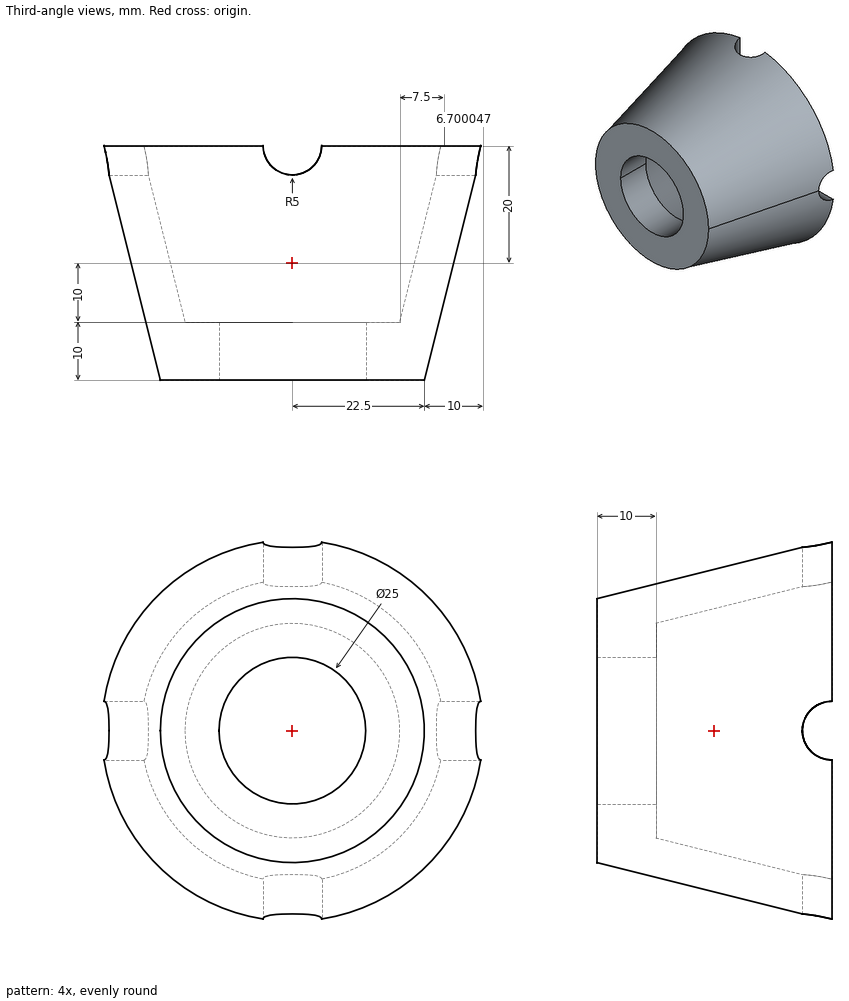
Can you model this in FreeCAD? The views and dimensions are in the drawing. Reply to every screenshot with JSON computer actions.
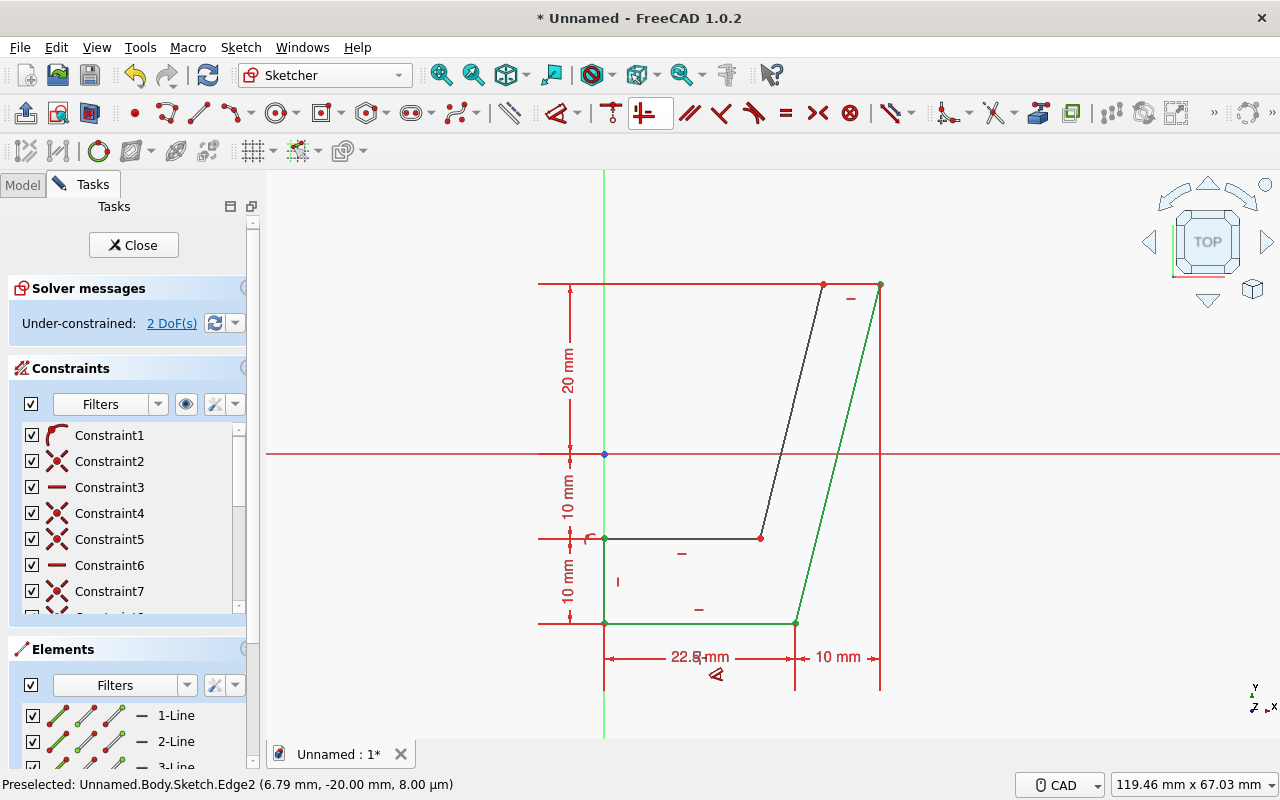
{"action": "left_click", "coordinate": [804, 361]}
{"action": "left_click", "coordinate": [792, 250]}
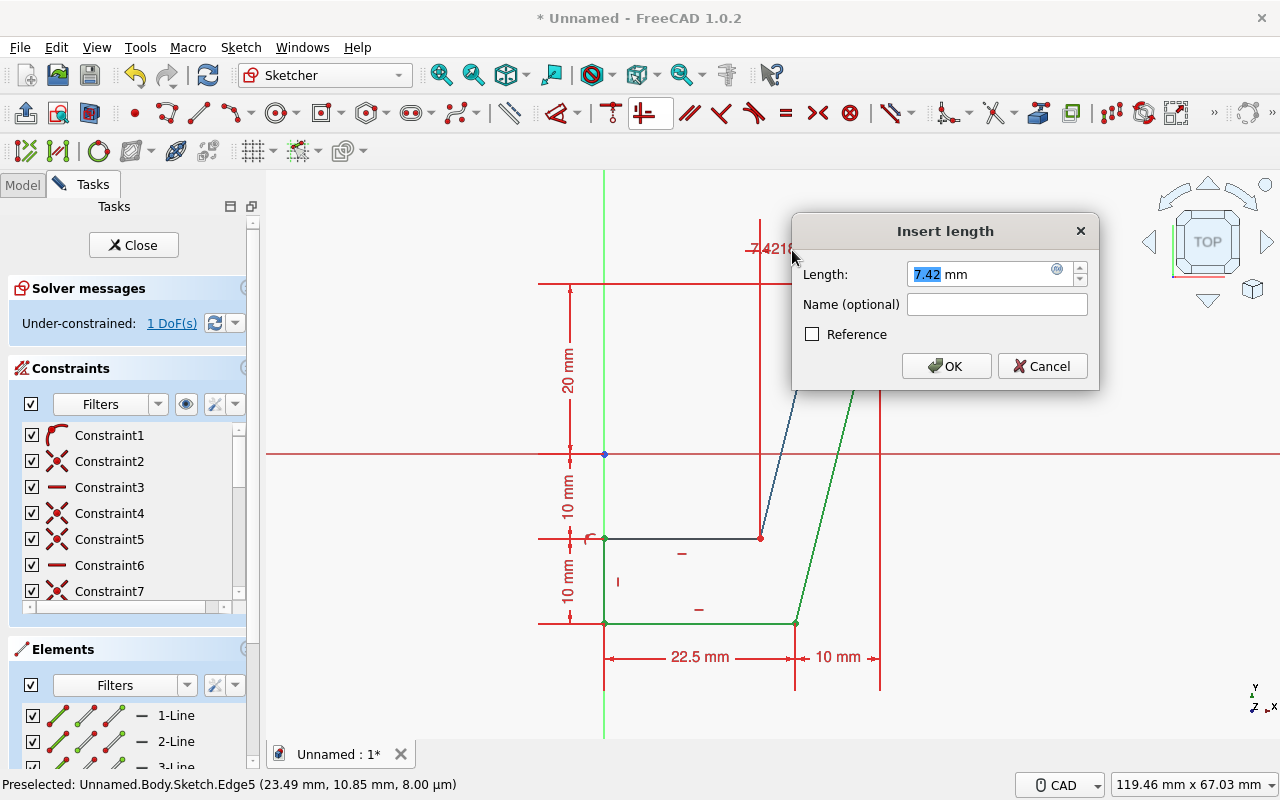
{"action": "type", "text": "7.5"}
{"action": "key", "text": "Return"}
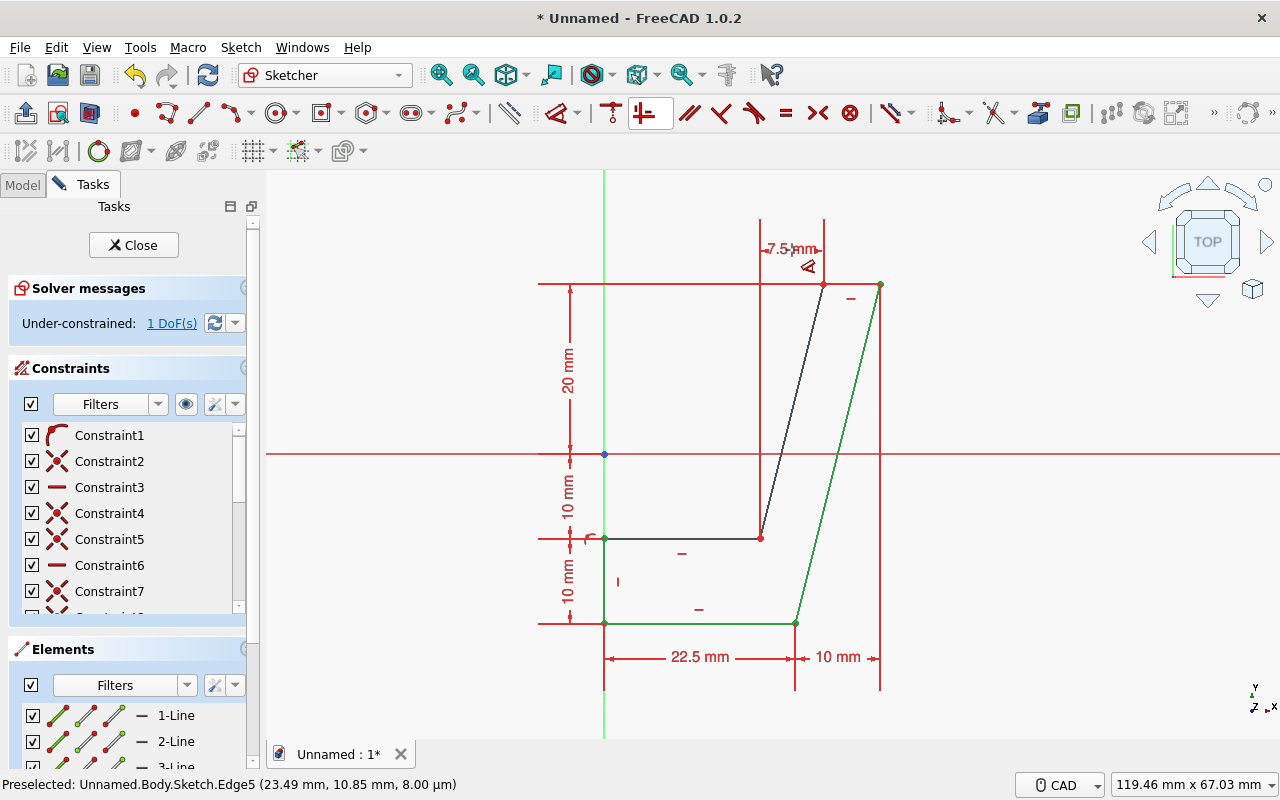
{"action": "left_click", "coordinate": [863, 284]}
{"action": "left_click", "coordinate": [865, 250]}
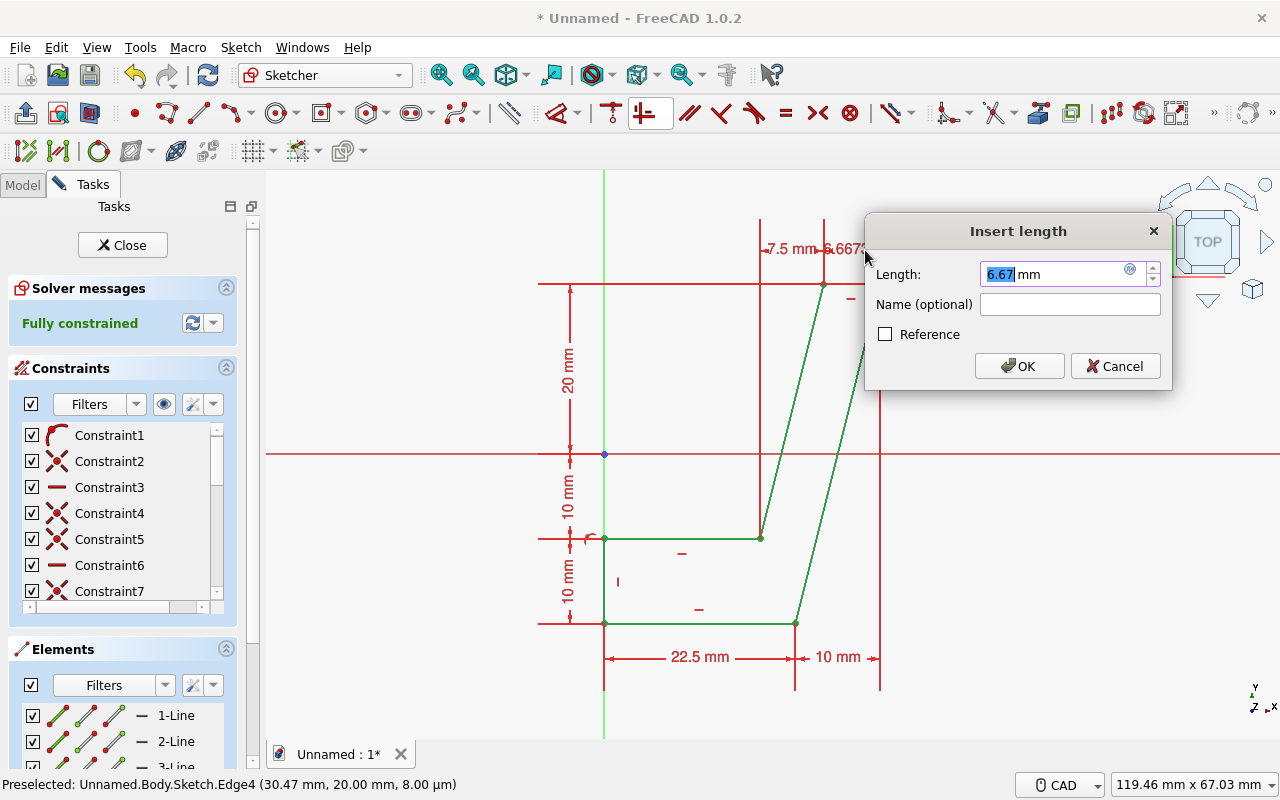
{"action": "type", "text": "6.700047"}
{"action": "key", "text": "Return"}
{"action": "key", "text": "Escape"}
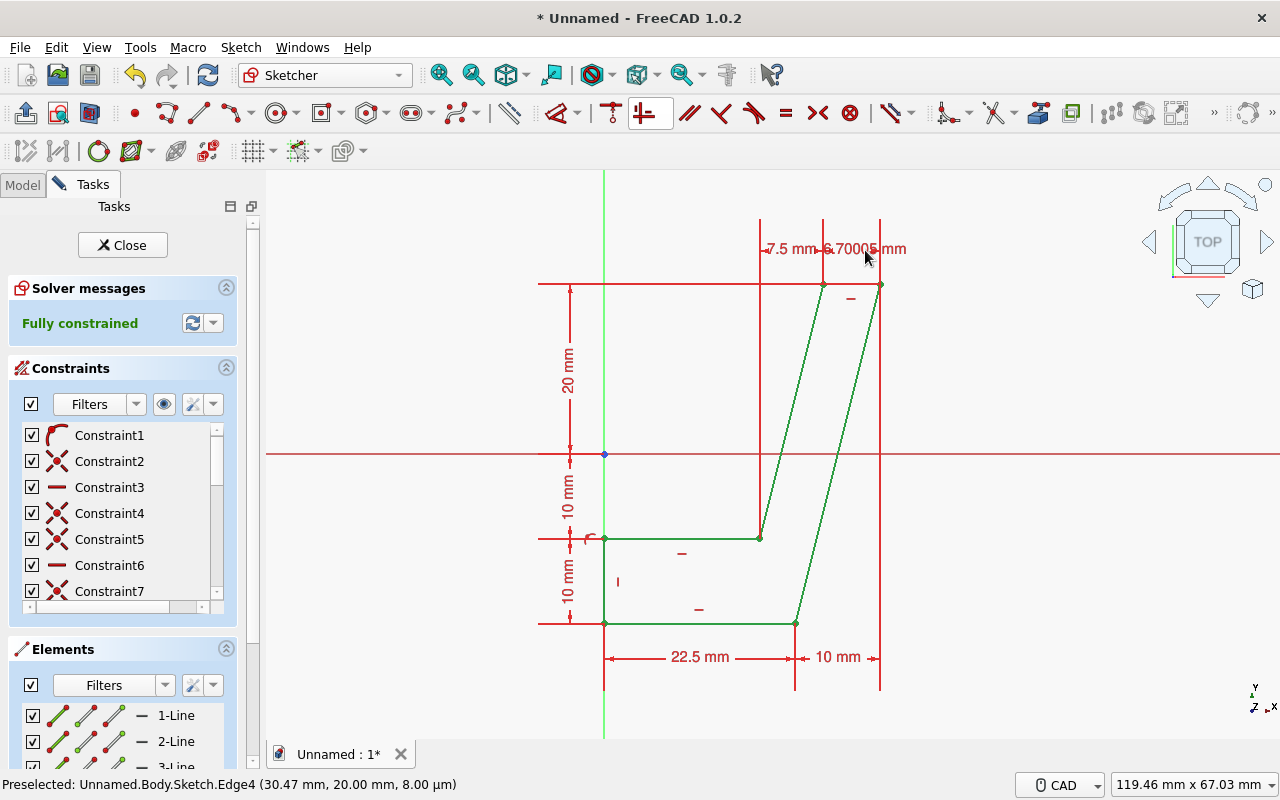
{"action": "left_click", "coordinate": [123, 245]}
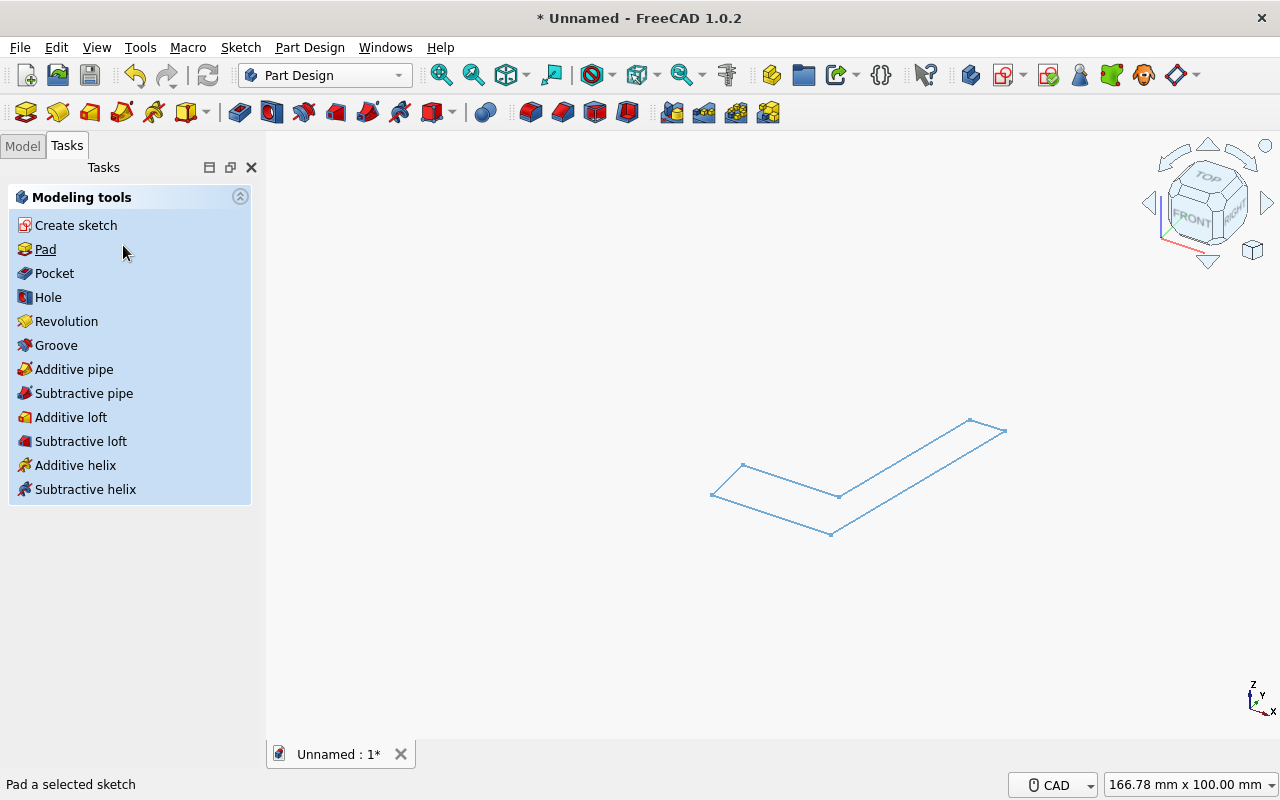
{"action": "left_click", "coordinate": [58, 112]}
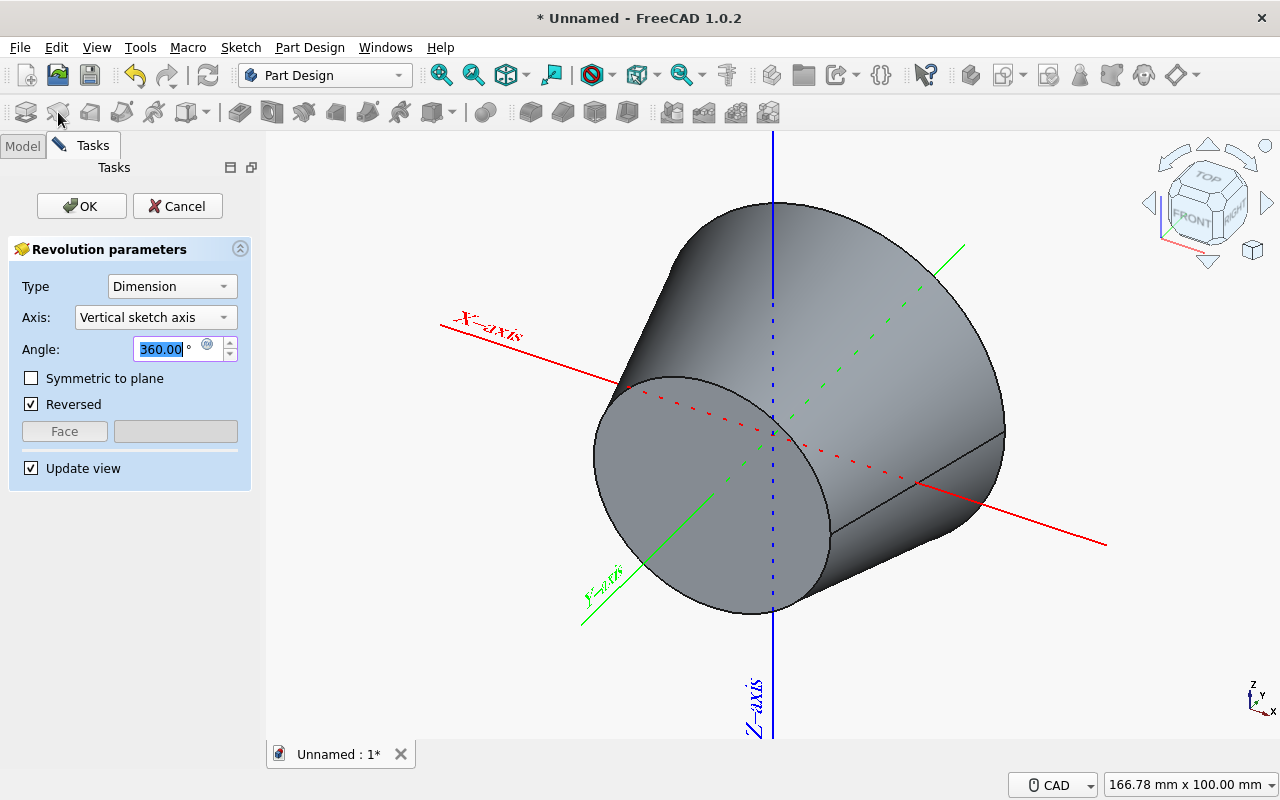
{"action": "left_click", "coordinate": [82, 206]}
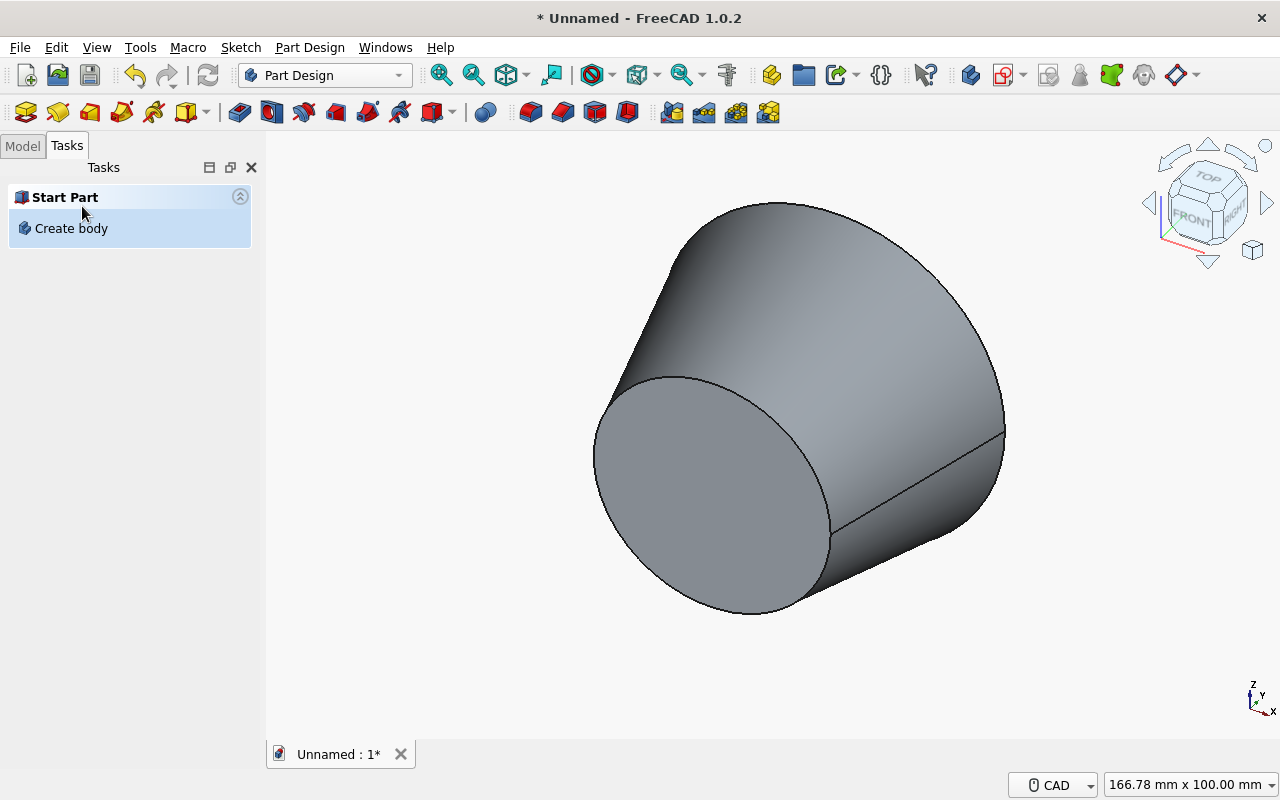
{"action": "key", "text": "4"}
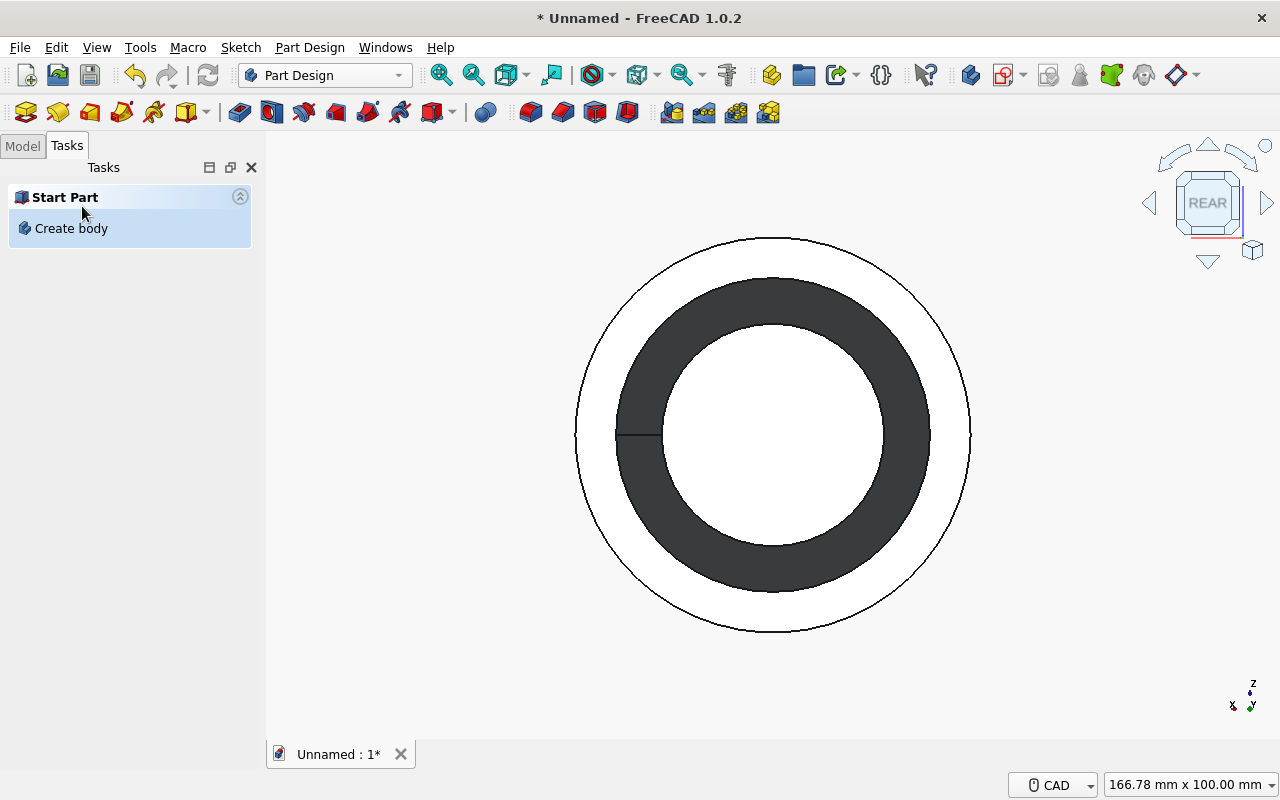
{"action": "left_click", "coordinate": [773, 434]}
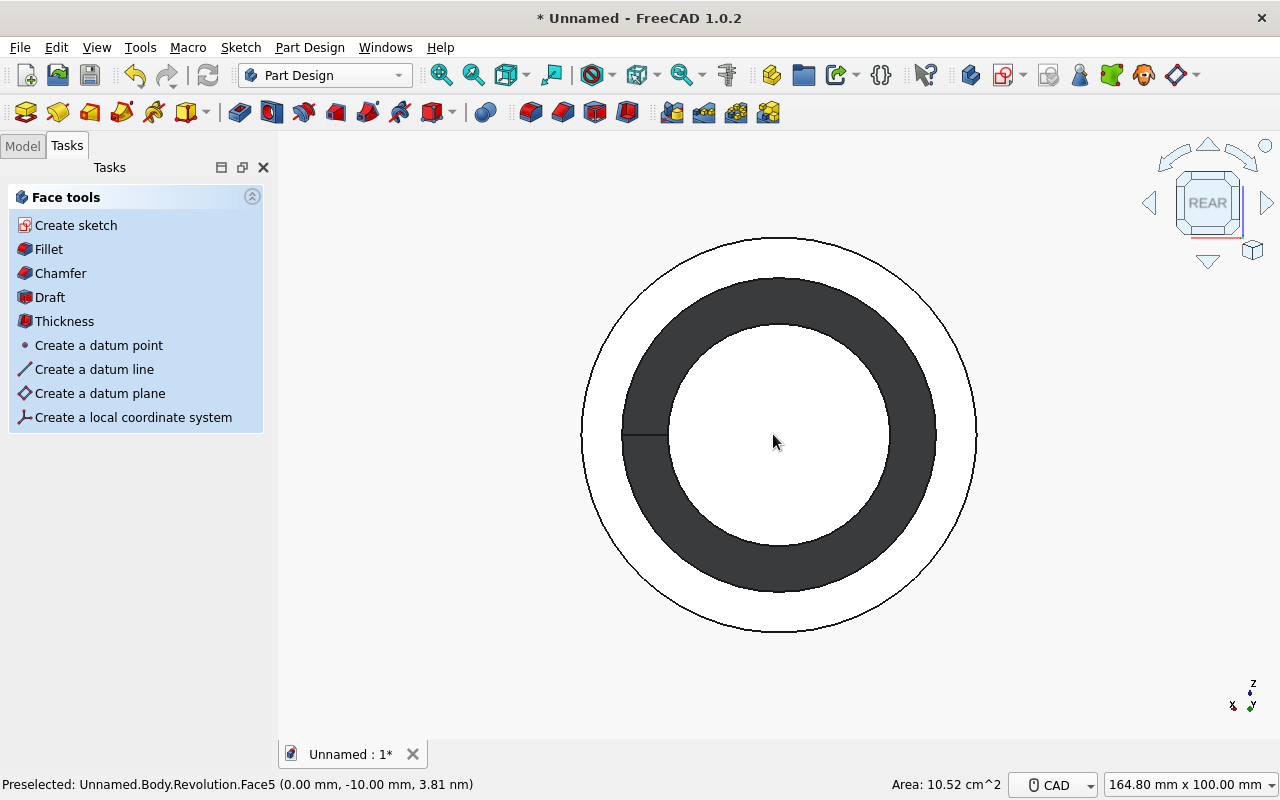
{"action": "left_click", "coordinate": [1004, 76]}